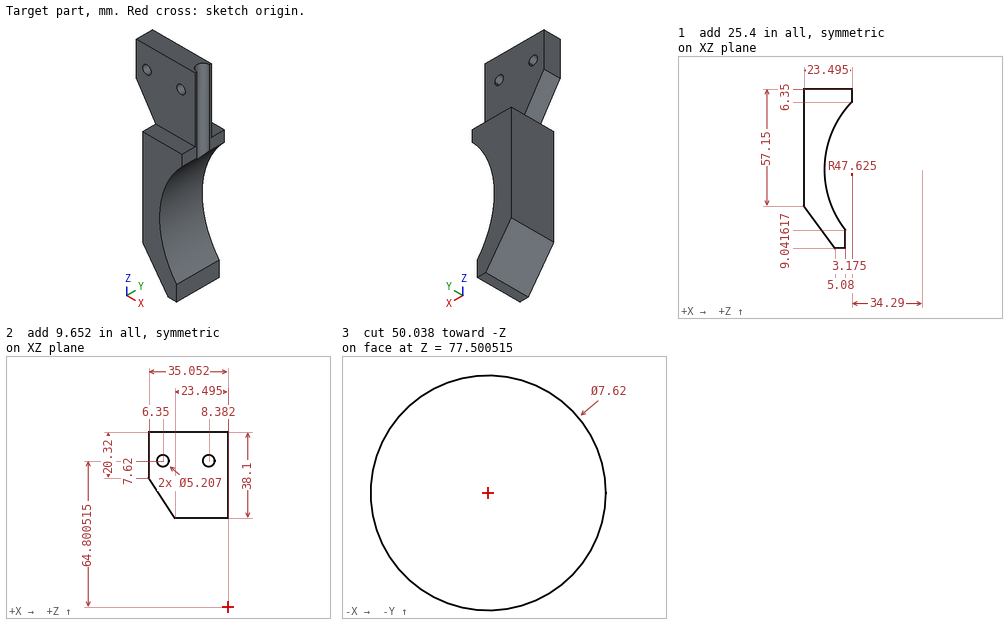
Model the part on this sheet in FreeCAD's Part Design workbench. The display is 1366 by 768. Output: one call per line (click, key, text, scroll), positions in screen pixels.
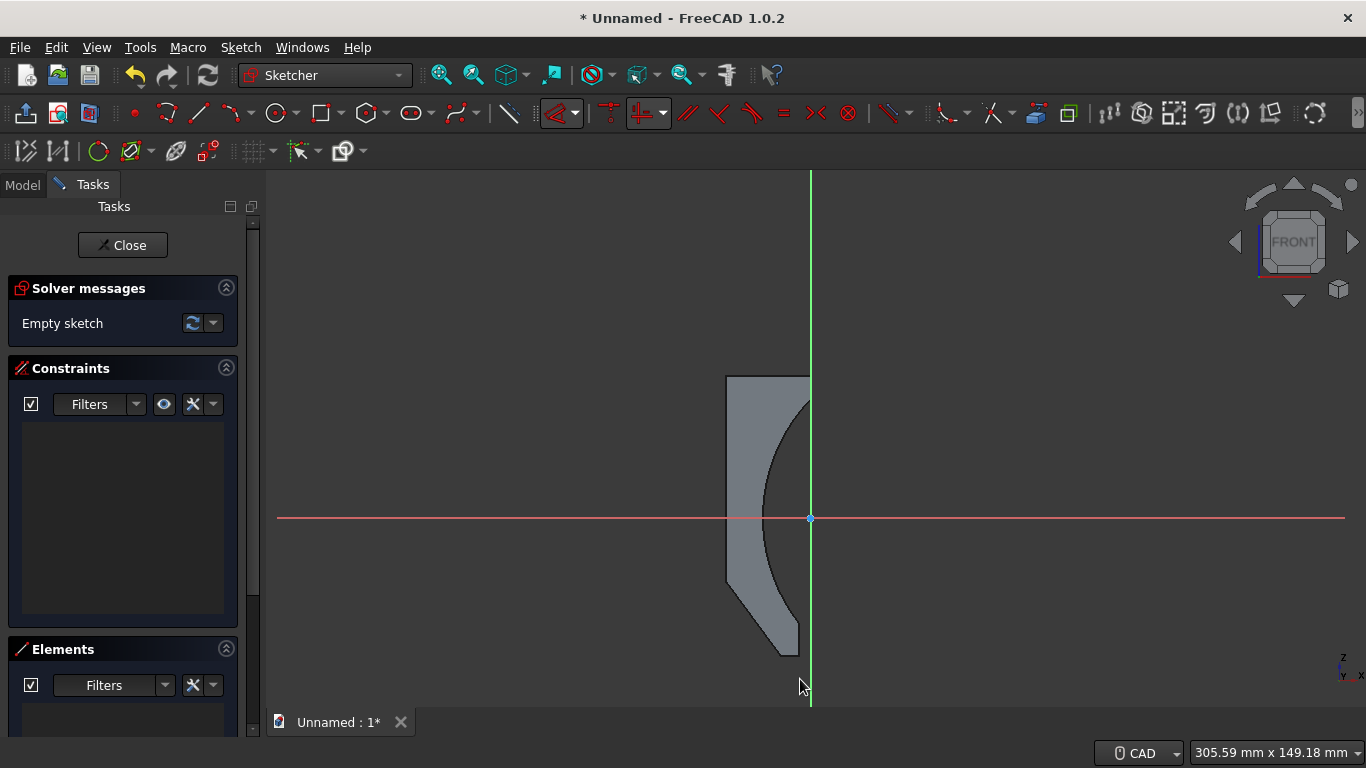
click(168, 114)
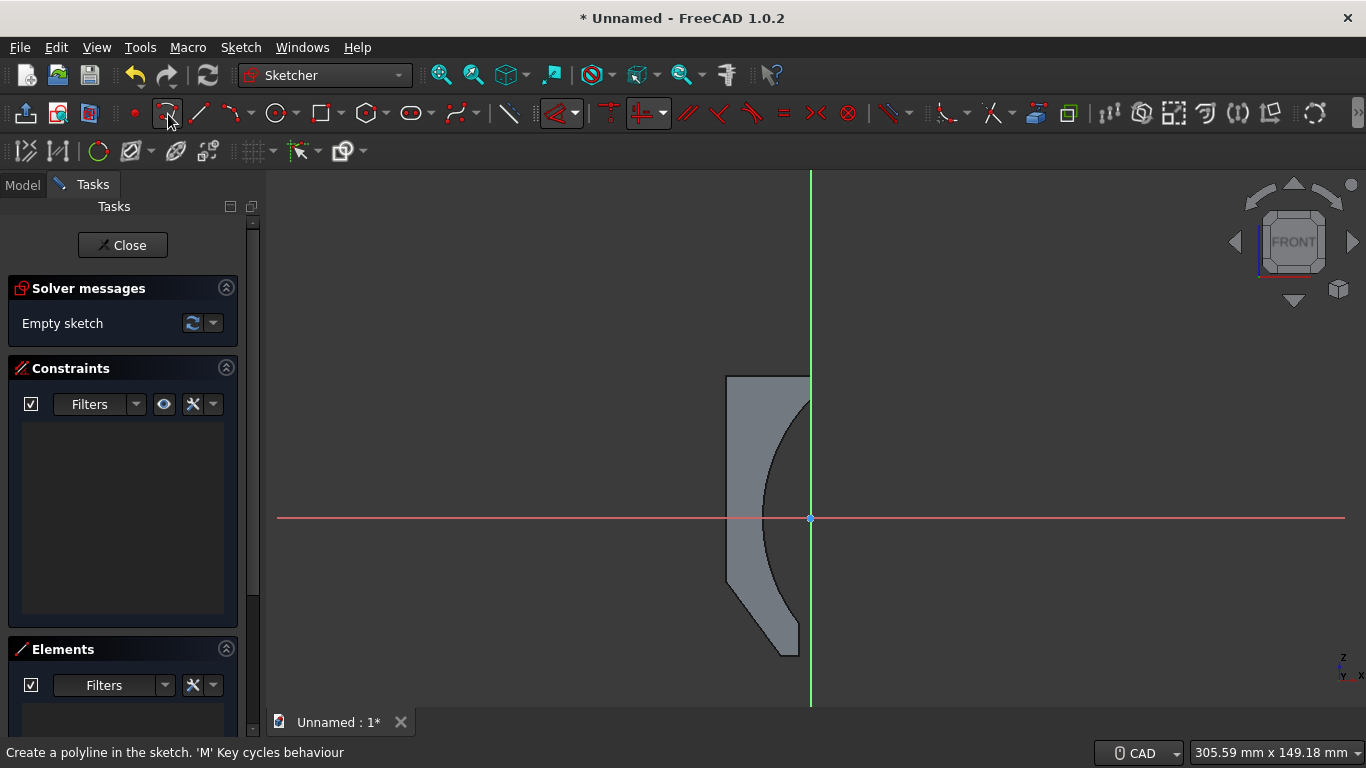
click(811, 376)
click(726, 376)
click(685, 312)
click(685, 239)
click(802, 239)
click(811, 377)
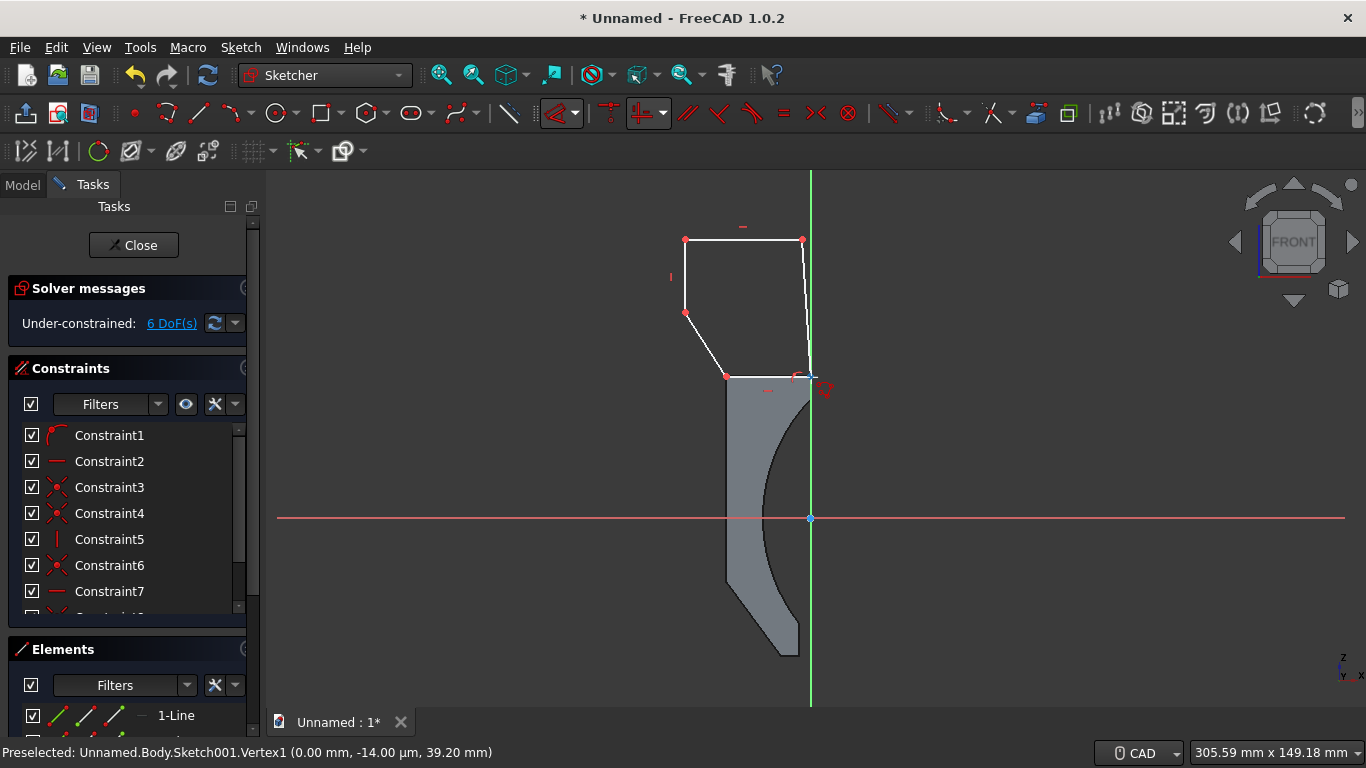
click(276, 114)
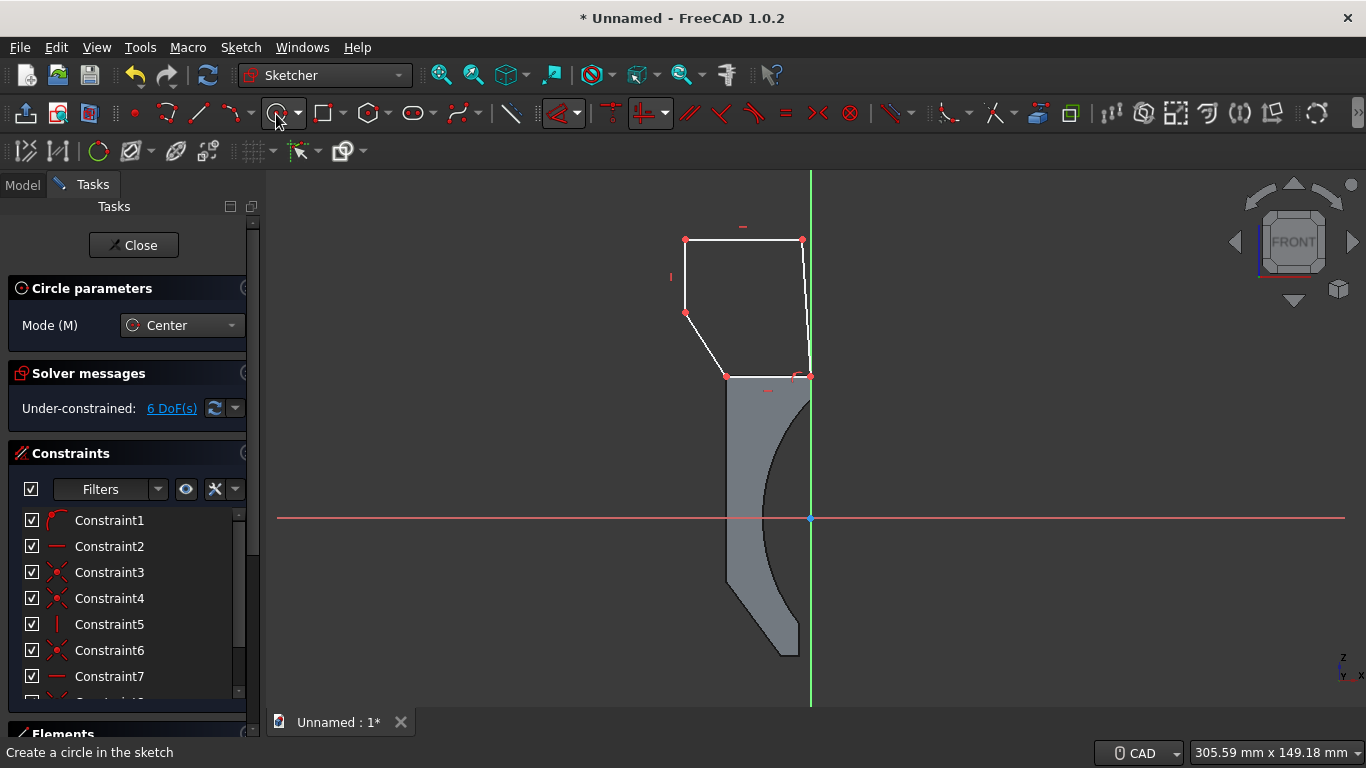
scroll(708, 285, up, 5)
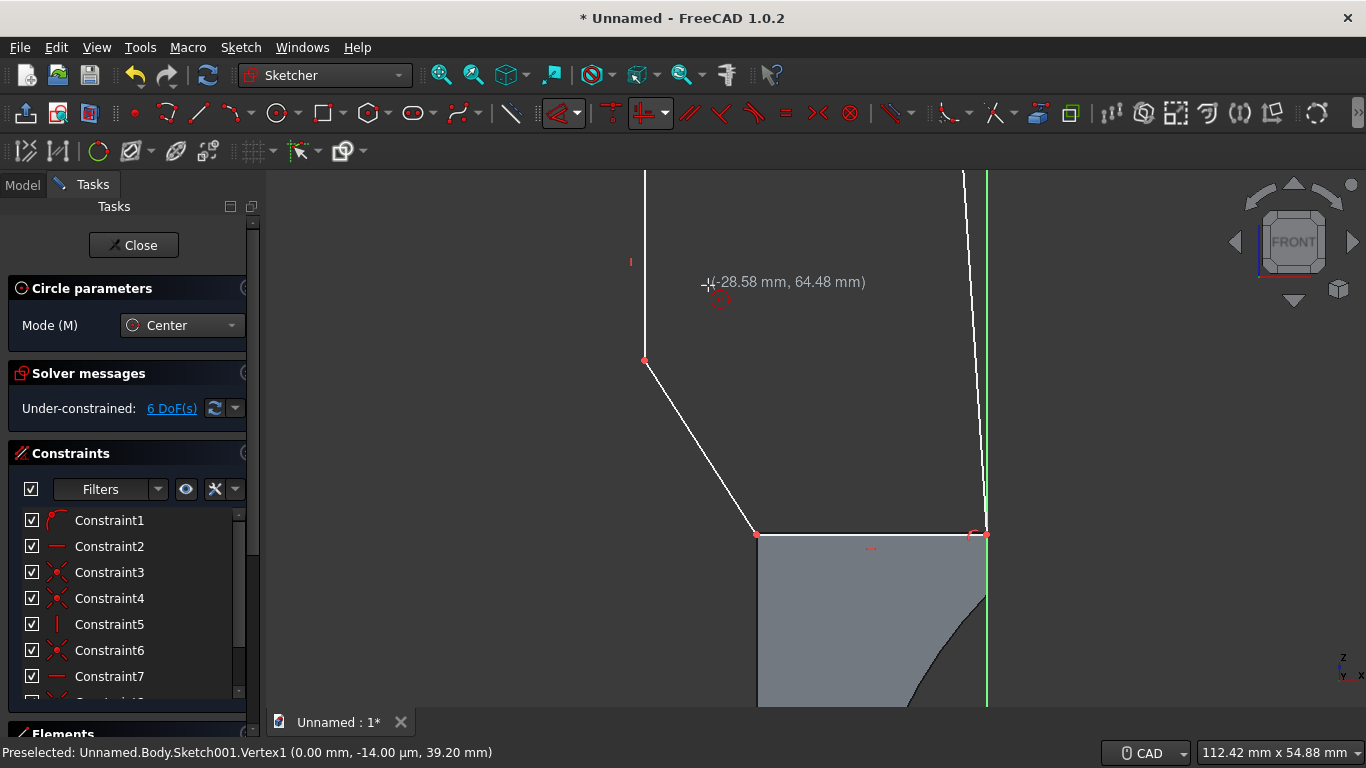
click(706, 284)
move(724, 266)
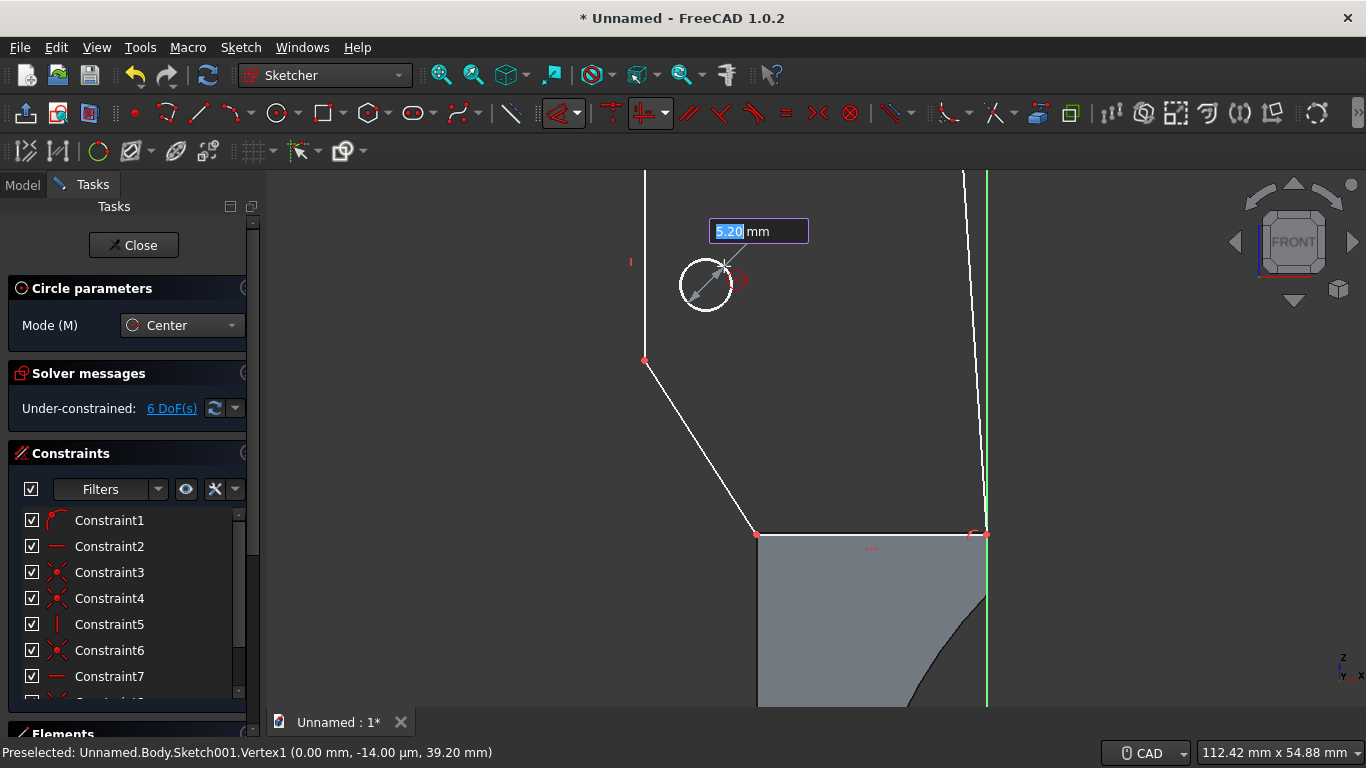
text(5.207)
key(Return)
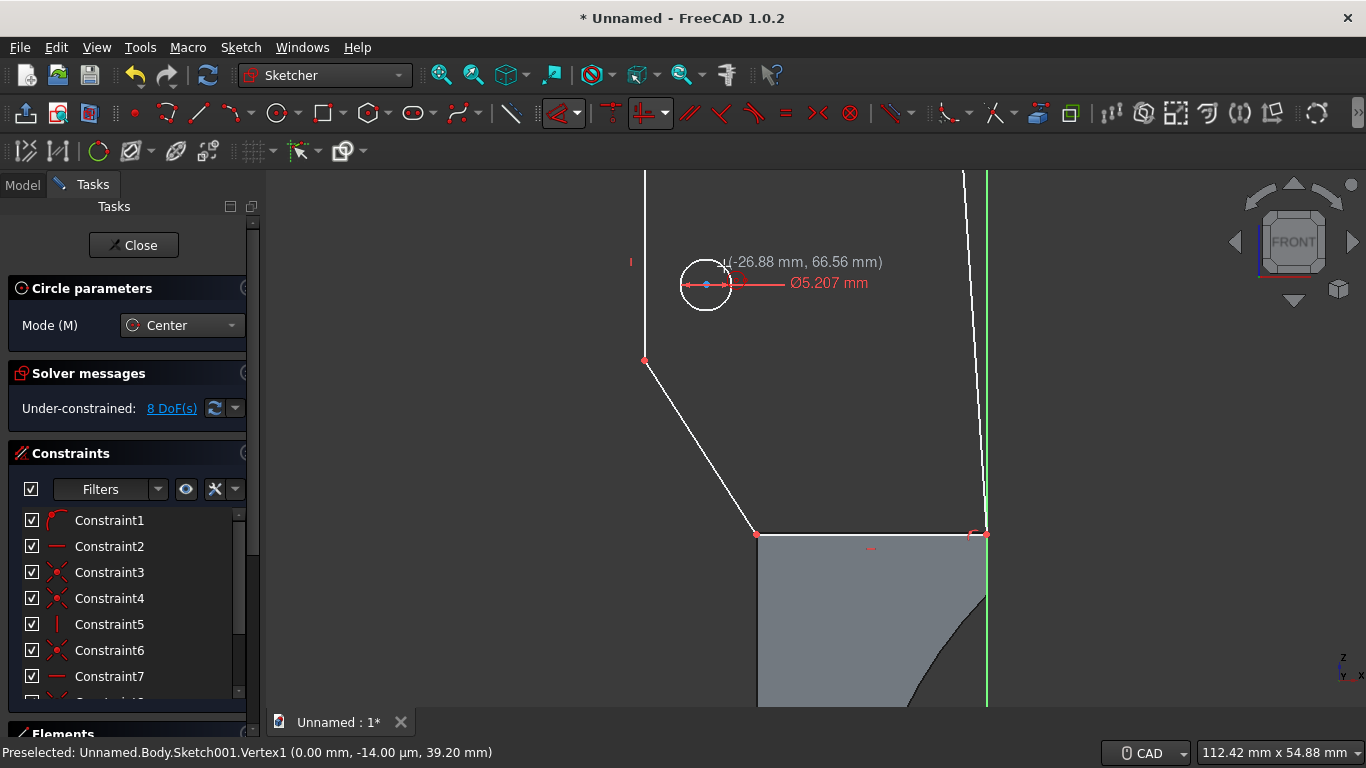
click(905, 284)
move(923, 266)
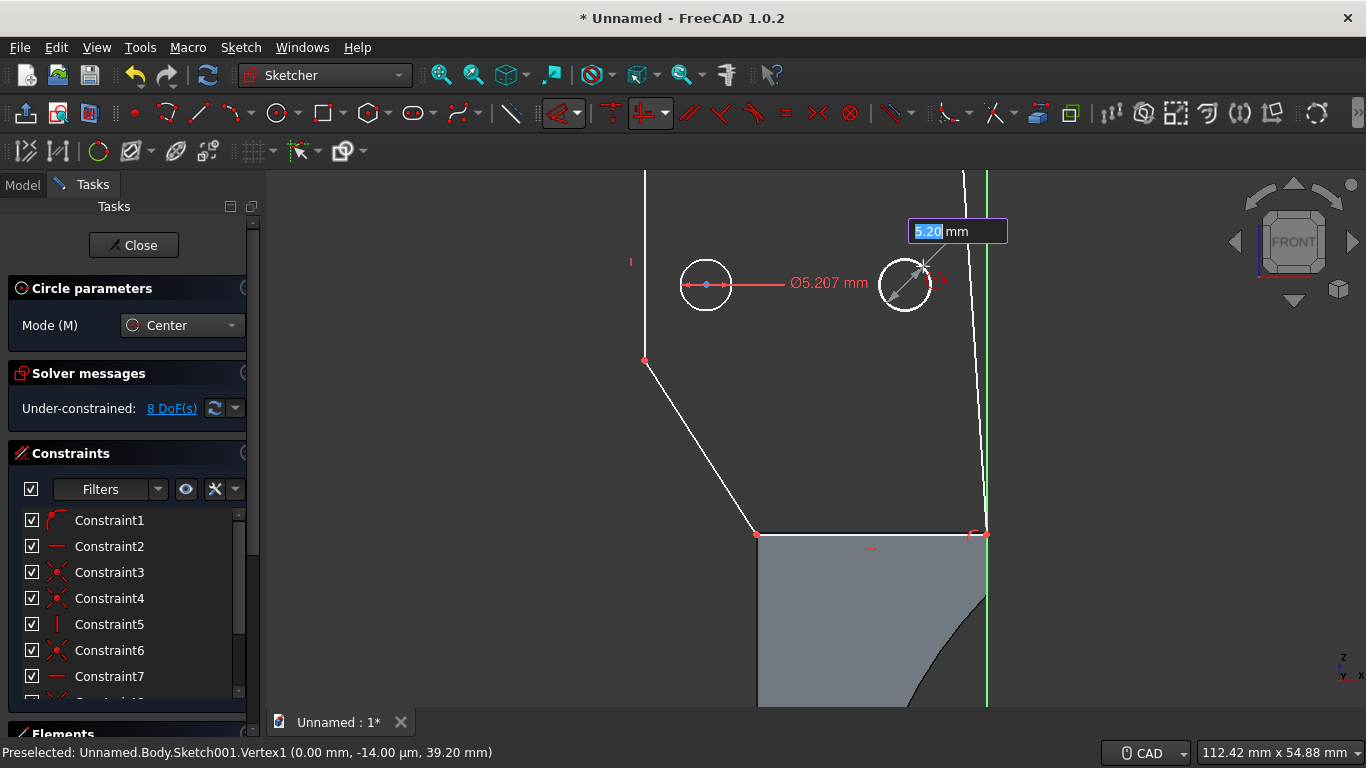
text(5.207)
key(Return)
key(Escape)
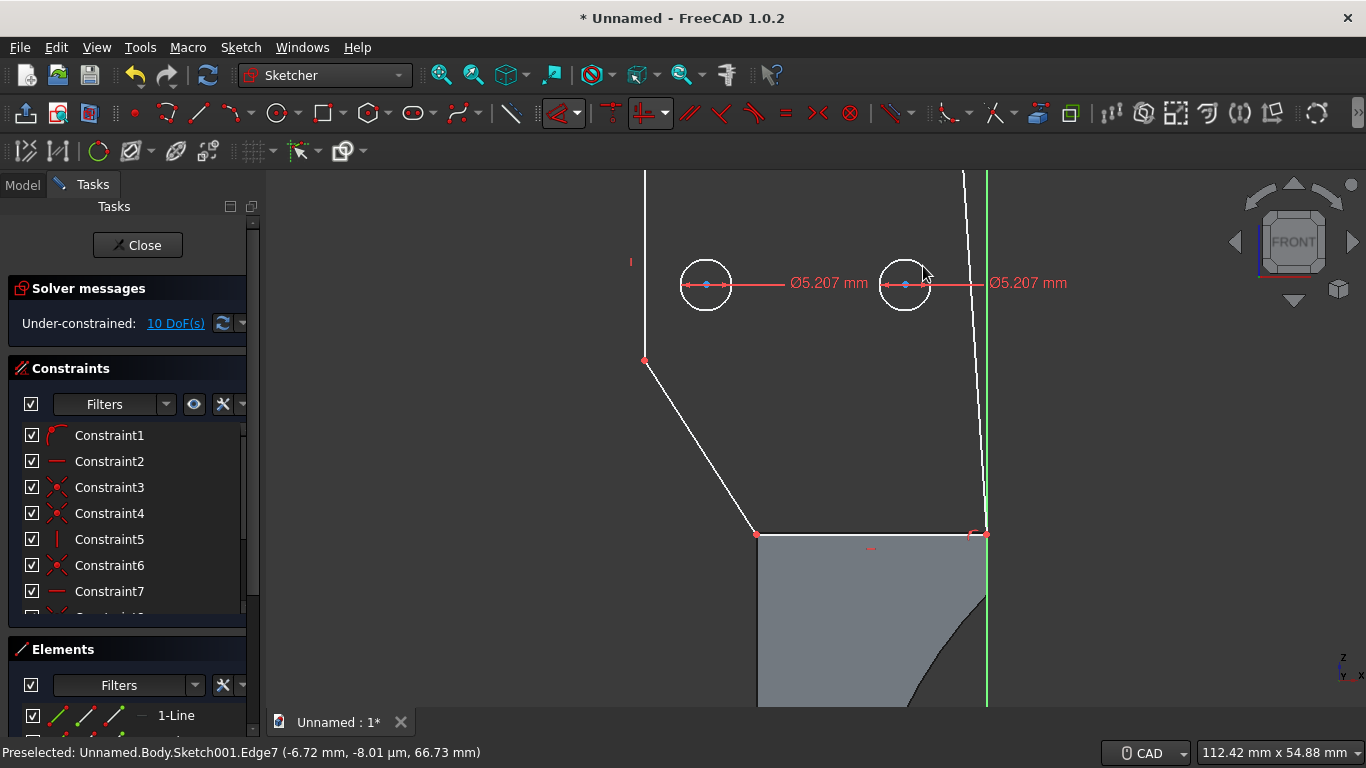
click(970, 274)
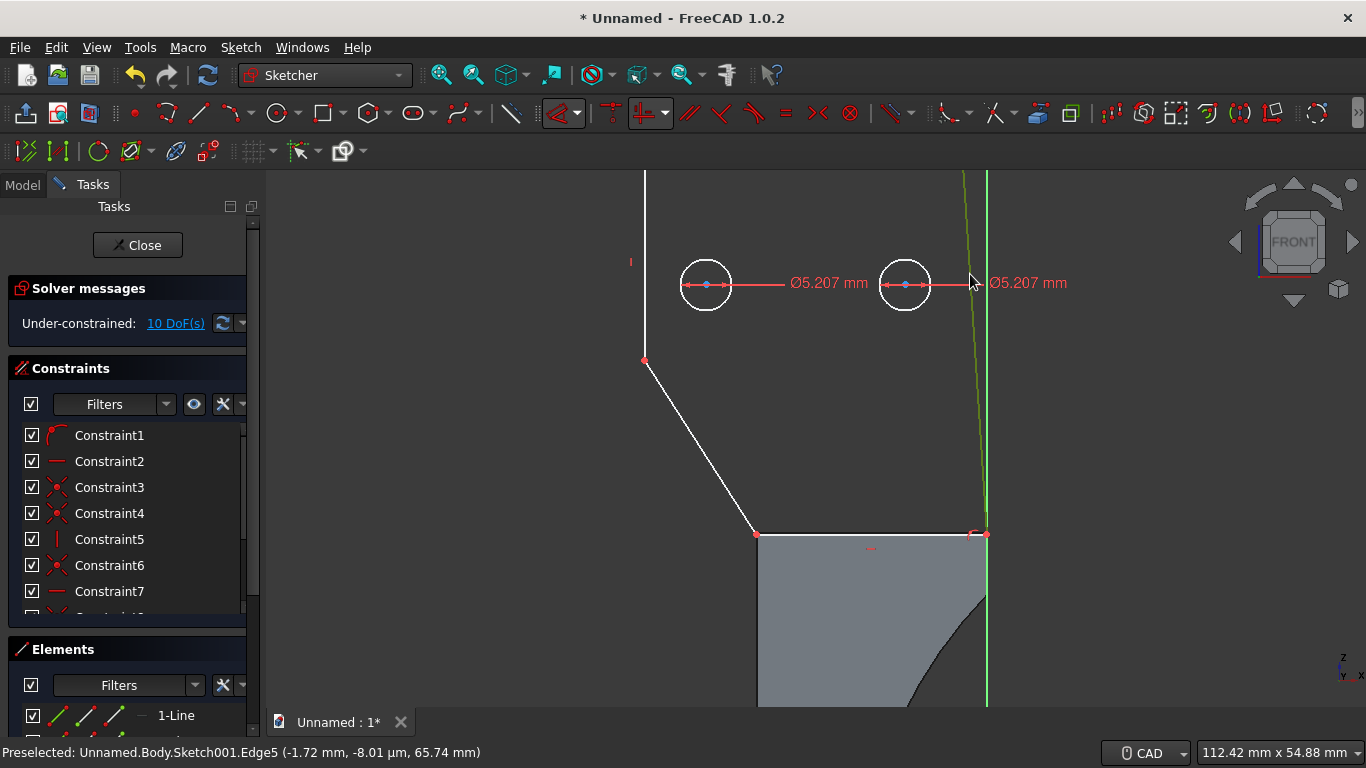
click(668, 114)